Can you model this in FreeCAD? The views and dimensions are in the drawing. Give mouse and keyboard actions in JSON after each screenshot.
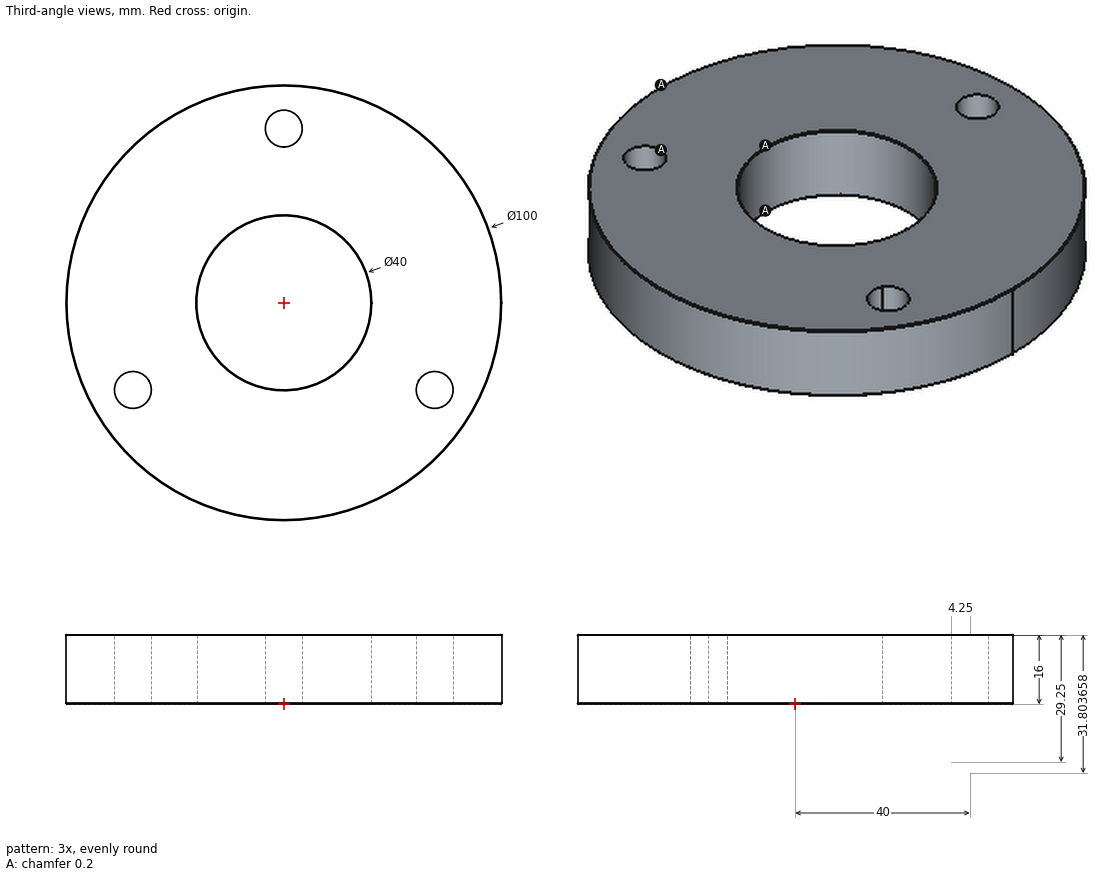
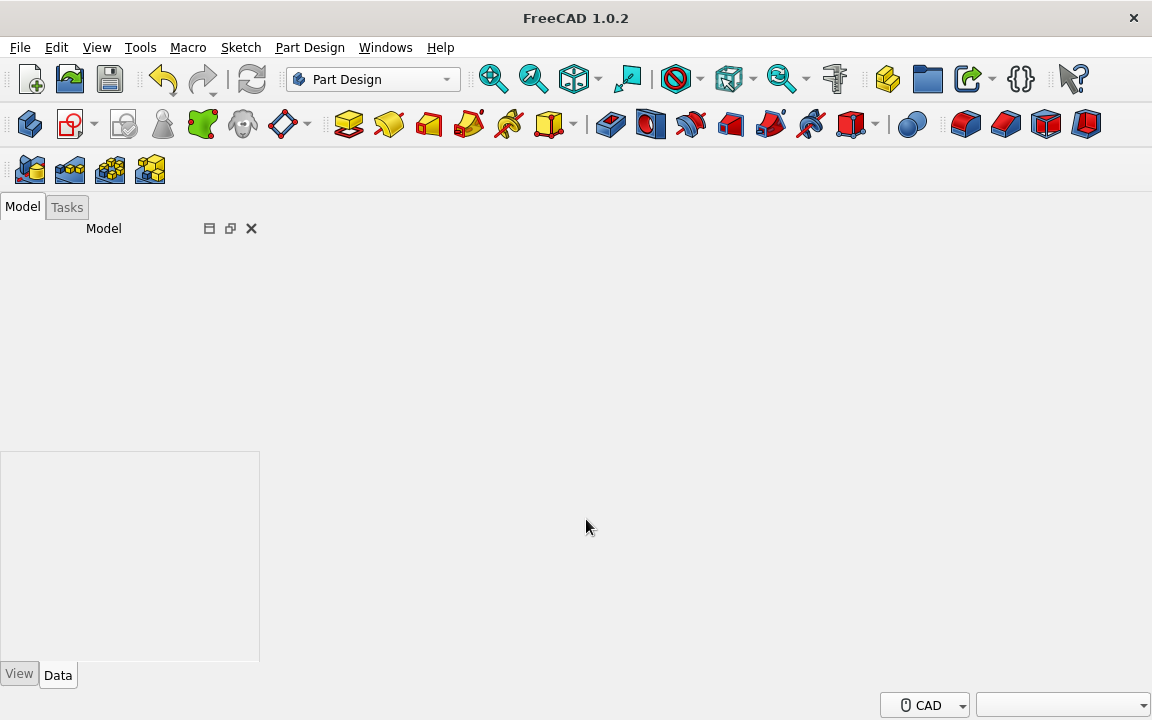
{"action": "left_click", "coordinate": [30, 80]}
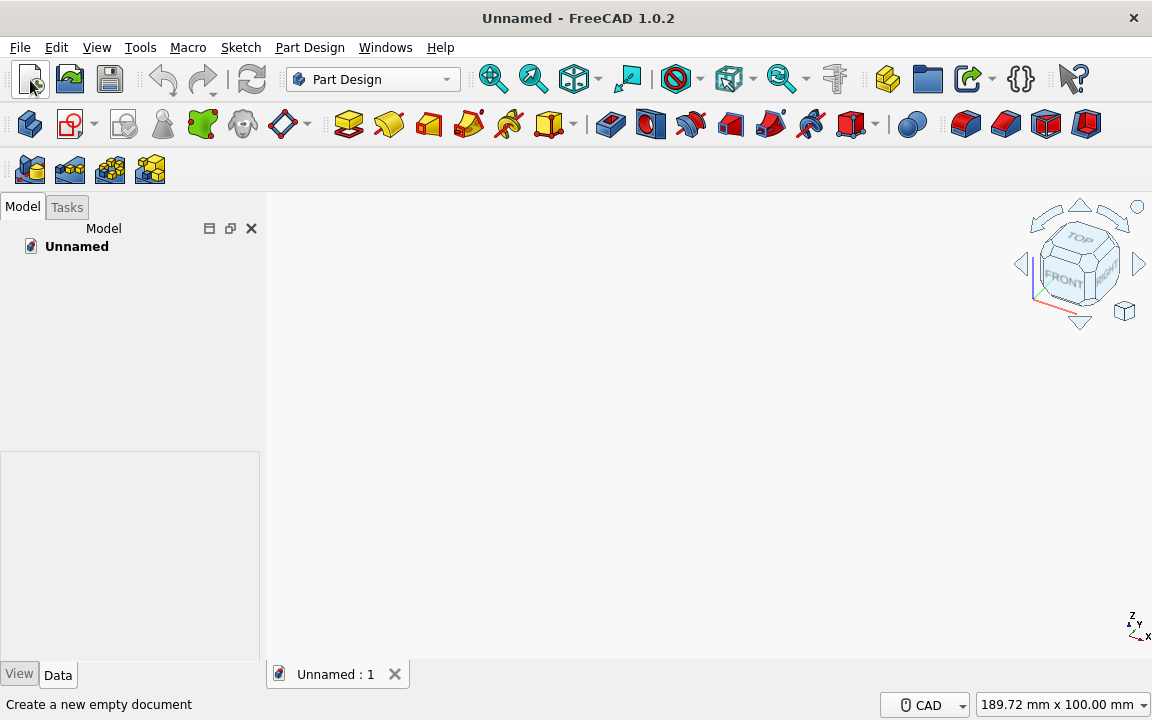
{"action": "left_click", "coordinate": [70, 124]}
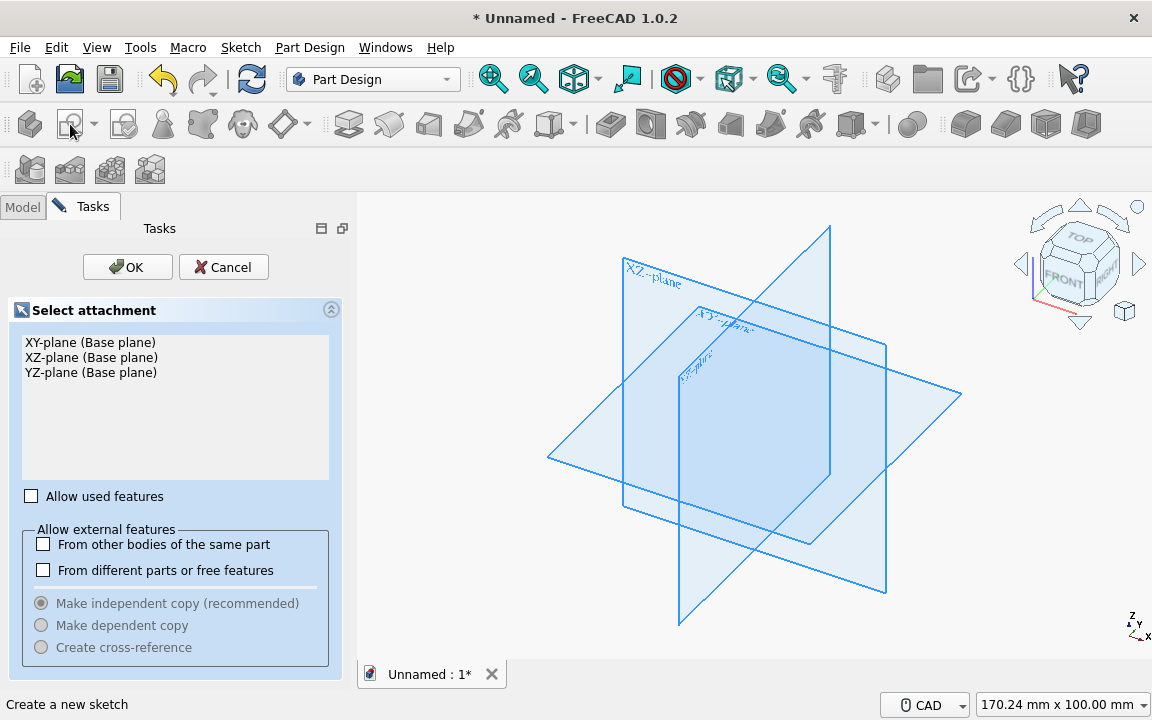
{"action": "left_click", "coordinate": [82, 342]}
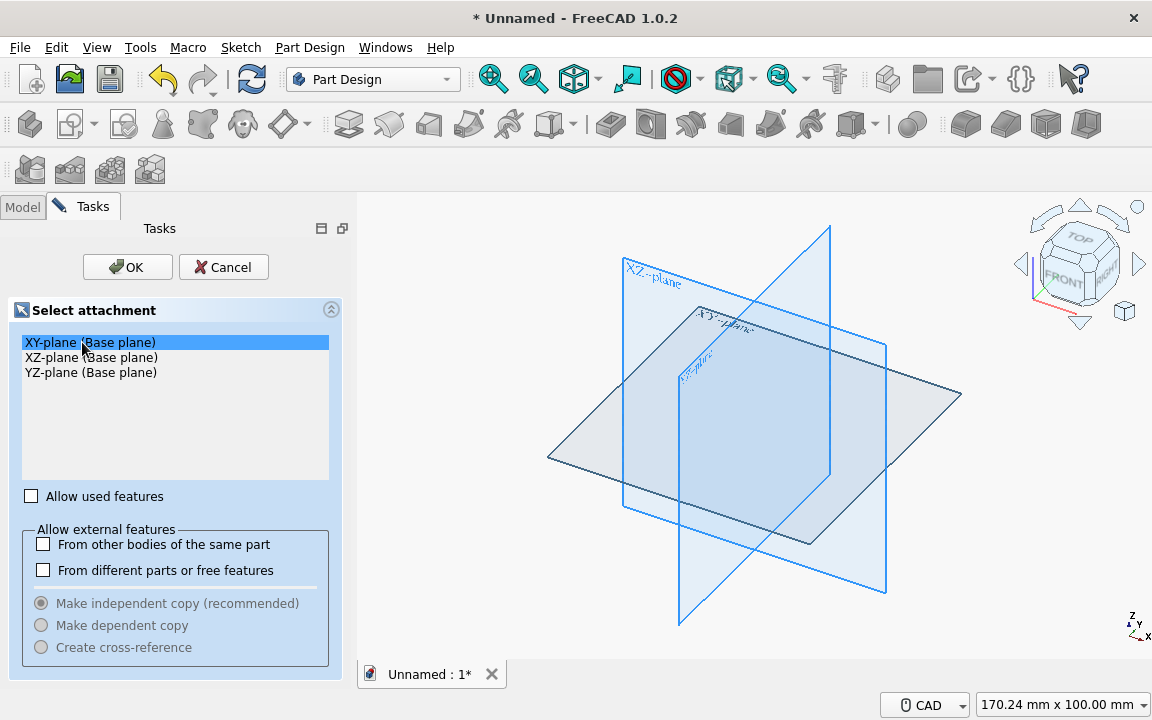
{"action": "left_click", "coordinate": [128, 267]}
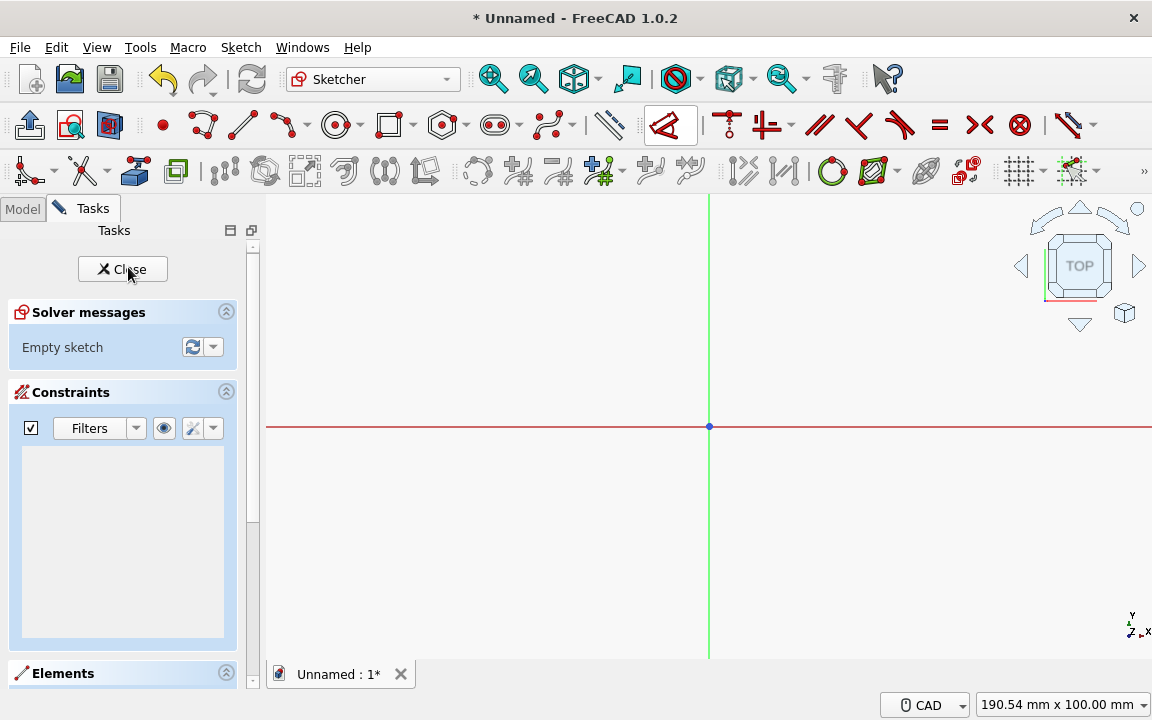
{"action": "scroll", "coordinate": [501, 427], "scroll_direction": "down", "scroll_amount": 2}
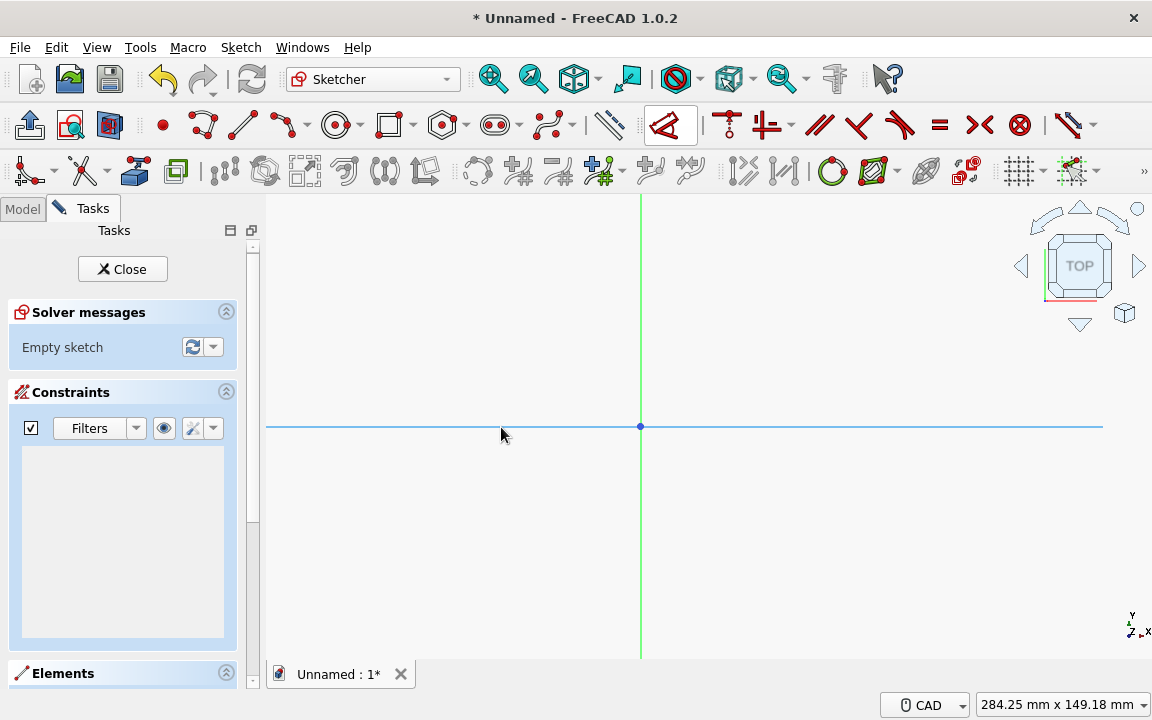
{"action": "left_click", "coordinate": [336, 126]}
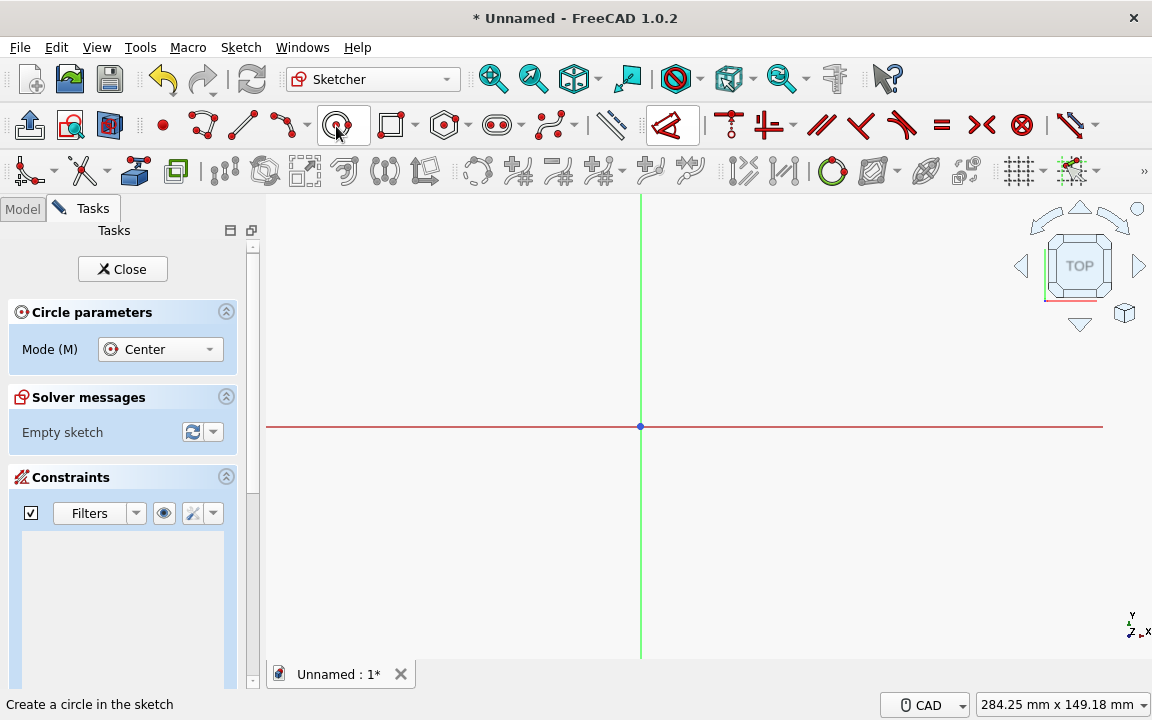
{"action": "left_click", "coordinate": [641, 427]}
{"action": "left_click", "coordinate": [751, 317]}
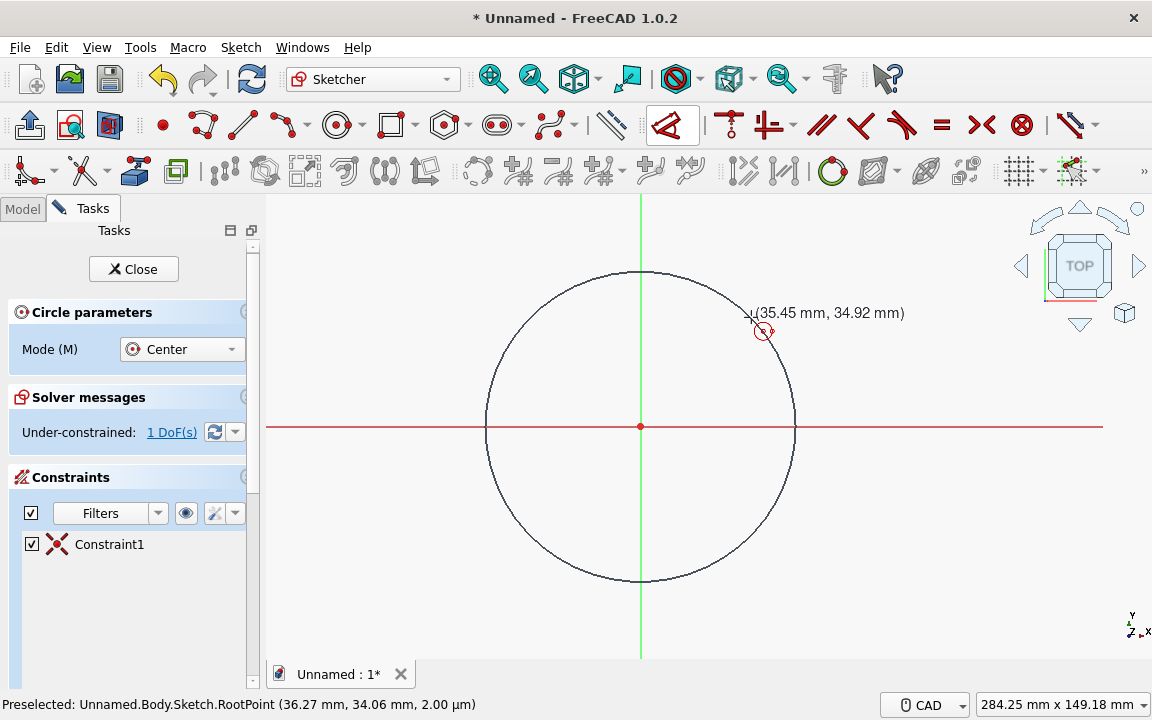
{"action": "left_click", "coordinate": [641, 427]}
{"action": "left_click", "coordinate": [685, 383]}
{"action": "key", "text": "Escape"}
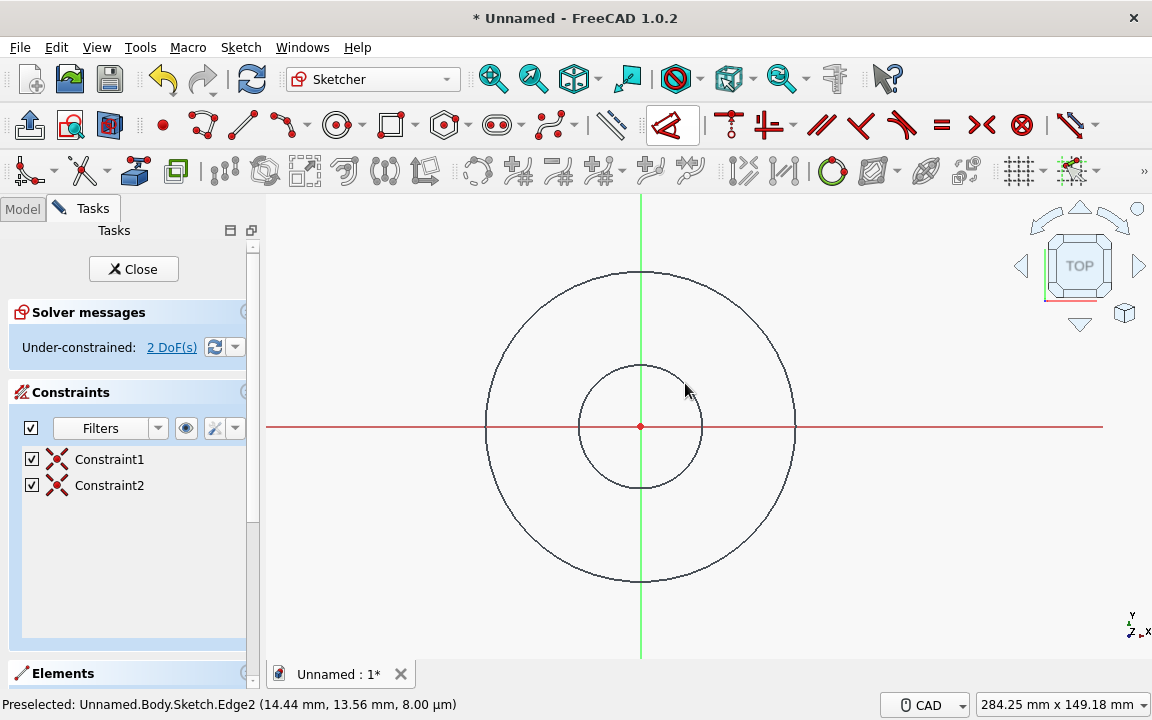
{"action": "left_click", "coordinate": [666, 126]}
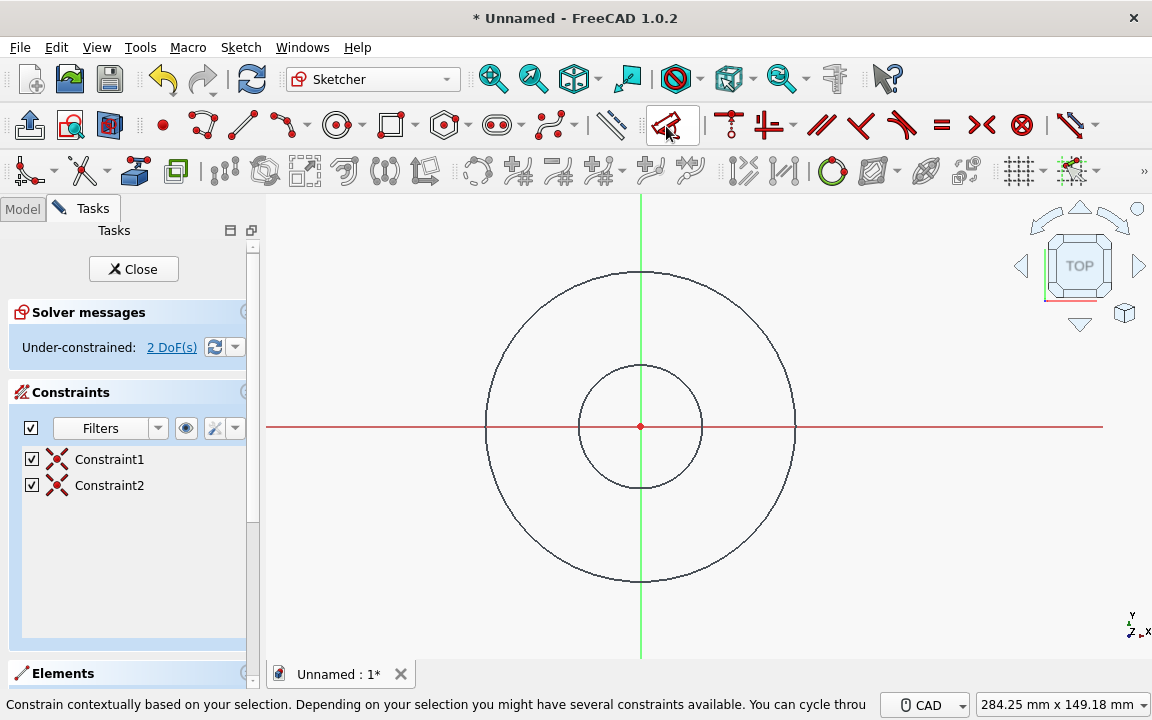
{"action": "left_click", "coordinate": [750, 317]}
{"action": "left_click", "coordinate": [773, 294]}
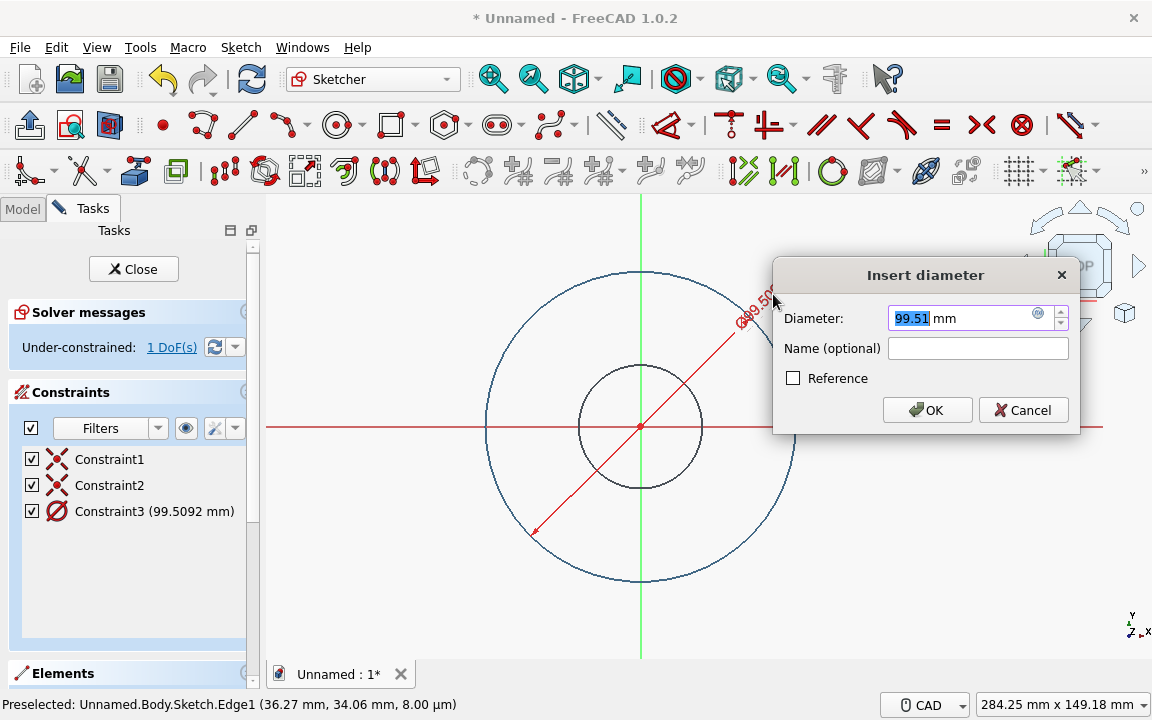
{"action": "type", "text": "100"}
{"action": "key", "text": "Return"}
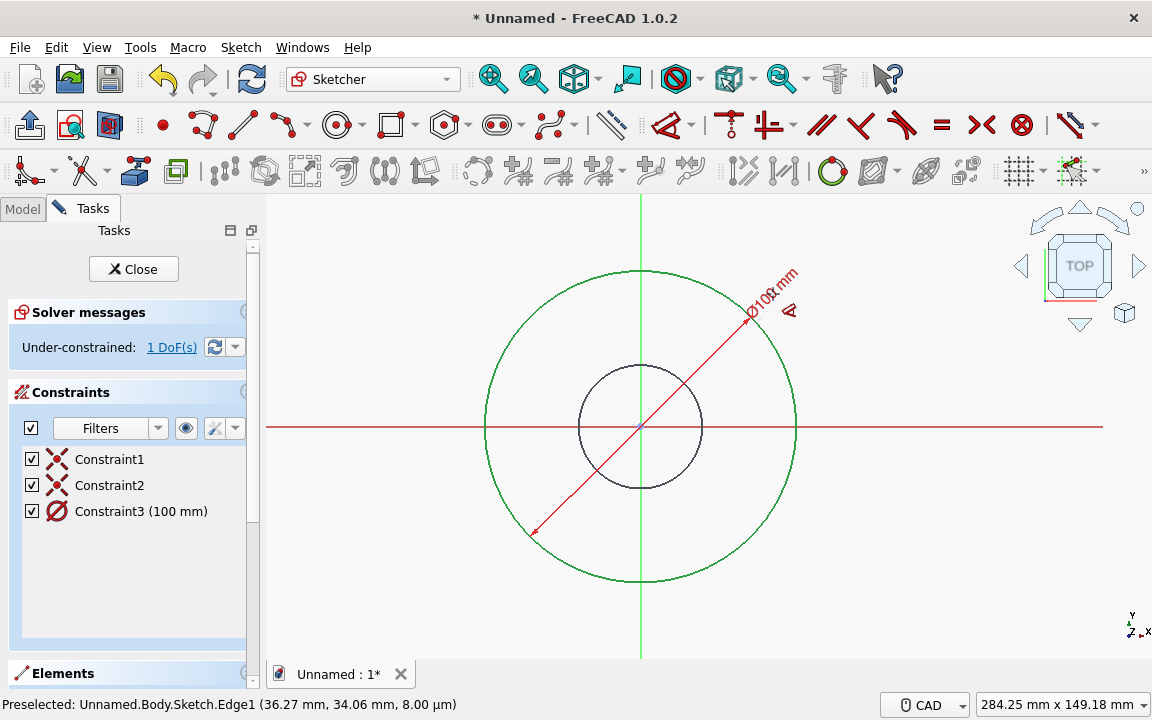
{"action": "left_click", "coordinate": [684, 383]}
{"action": "left_click", "coordinate": [707, 360]}